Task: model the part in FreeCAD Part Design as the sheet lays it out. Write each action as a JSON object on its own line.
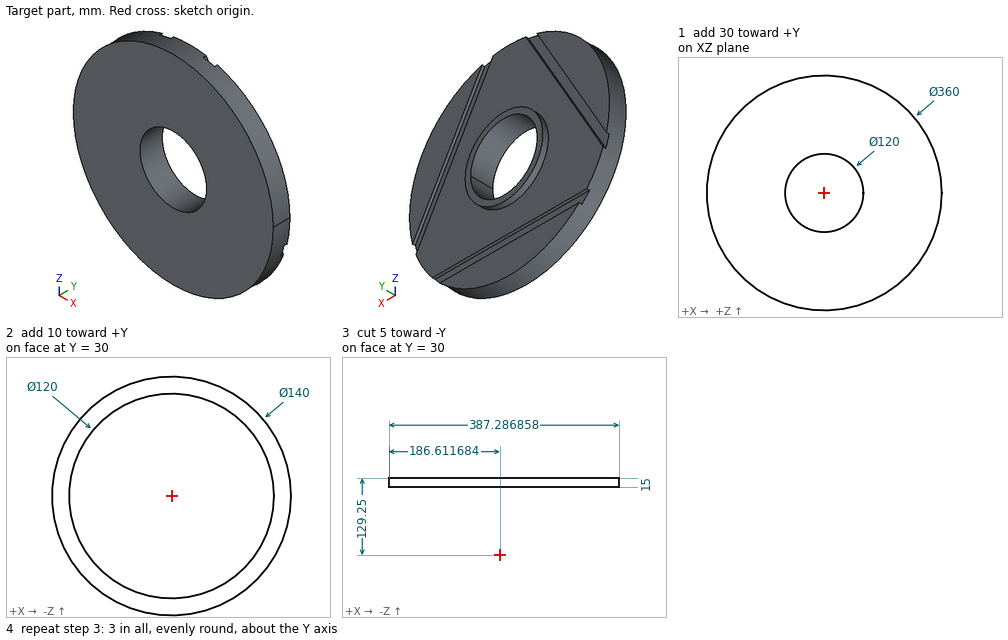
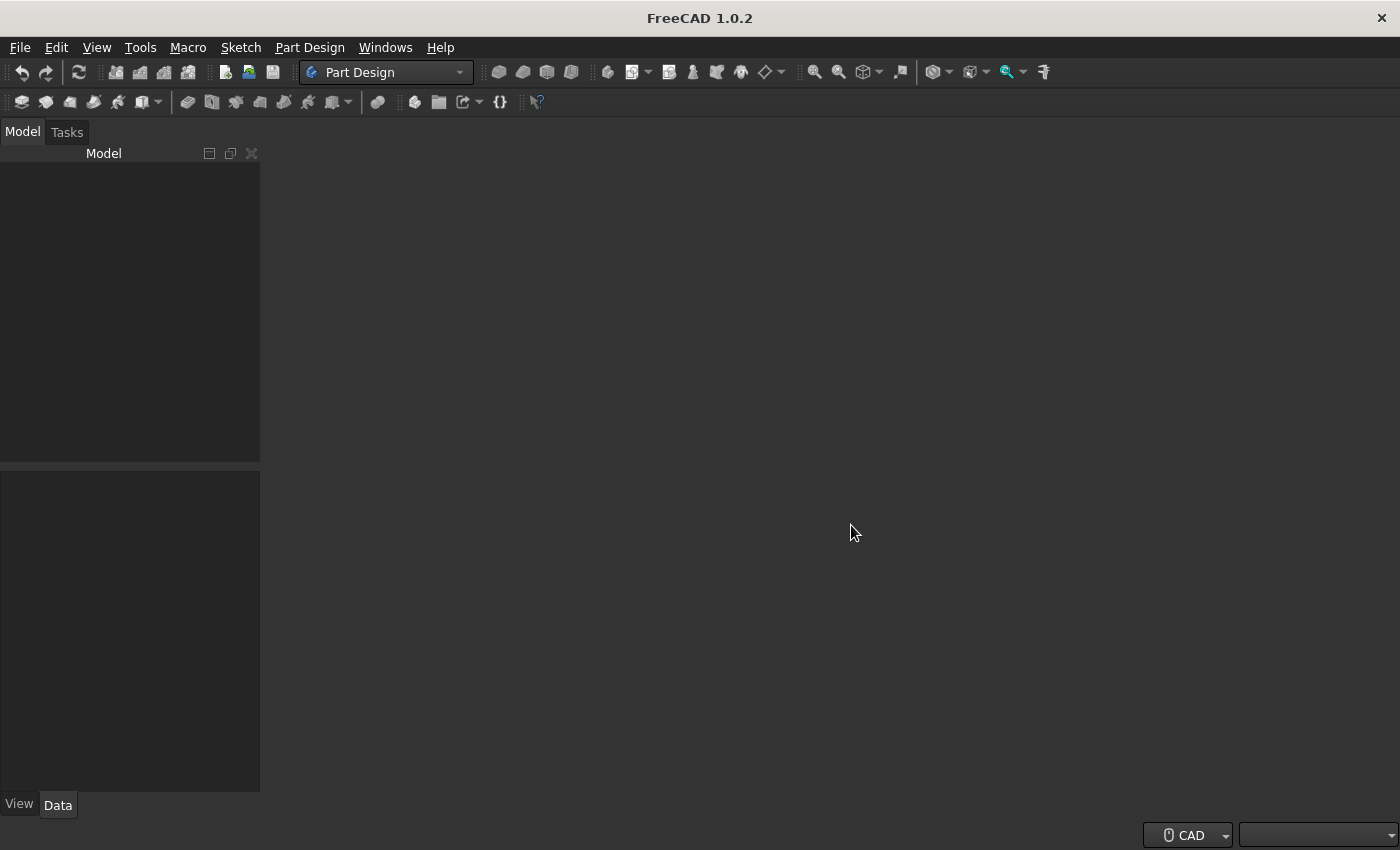
{"action": "left_click", "coordinate": [226, 72]}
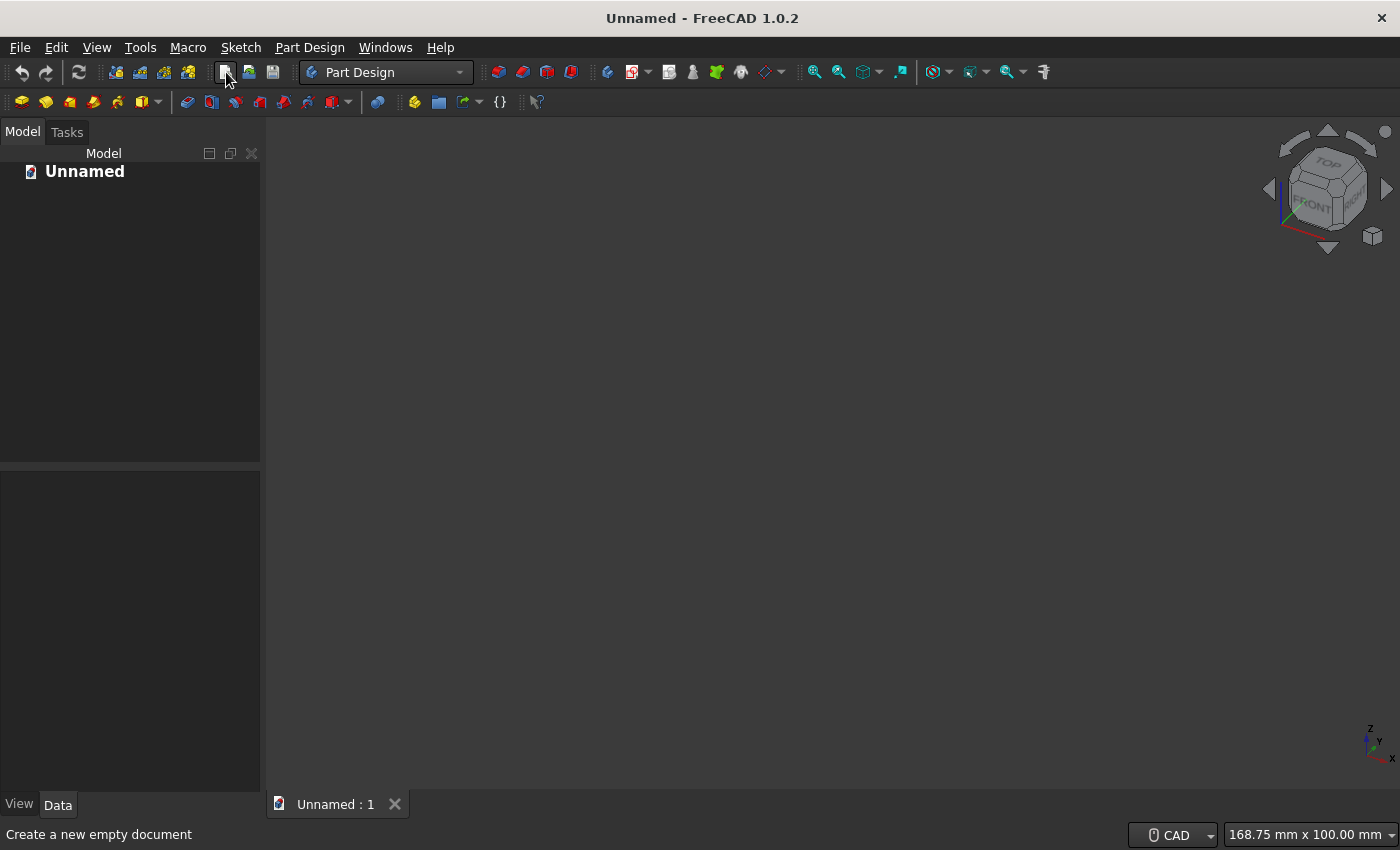
{"action": "left_click", "coordinate": [632, 72]}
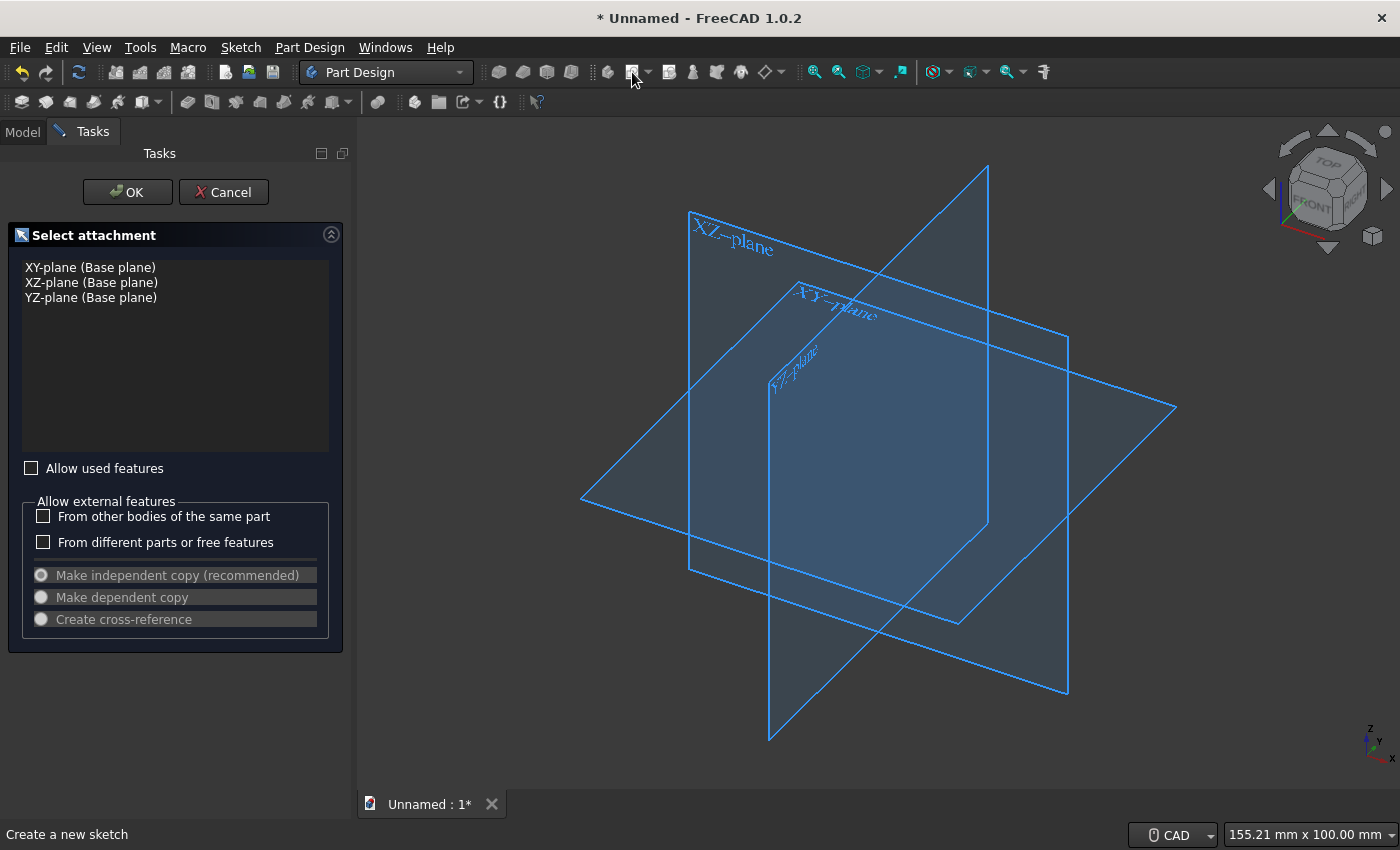
{"action": "left_click", "coordinate": [82, 282]}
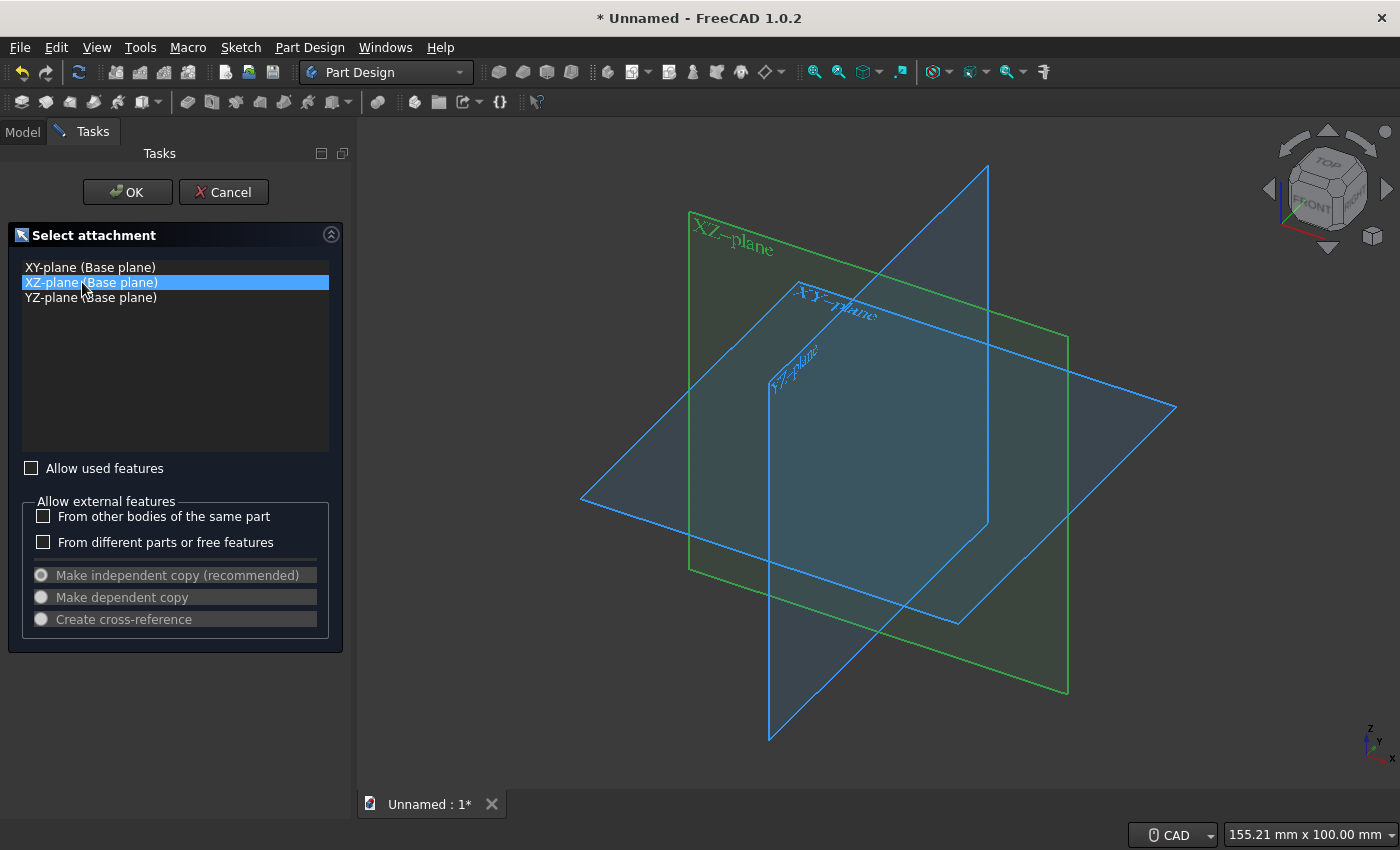
{"action": "left_click", "coordinate": [128, 192]}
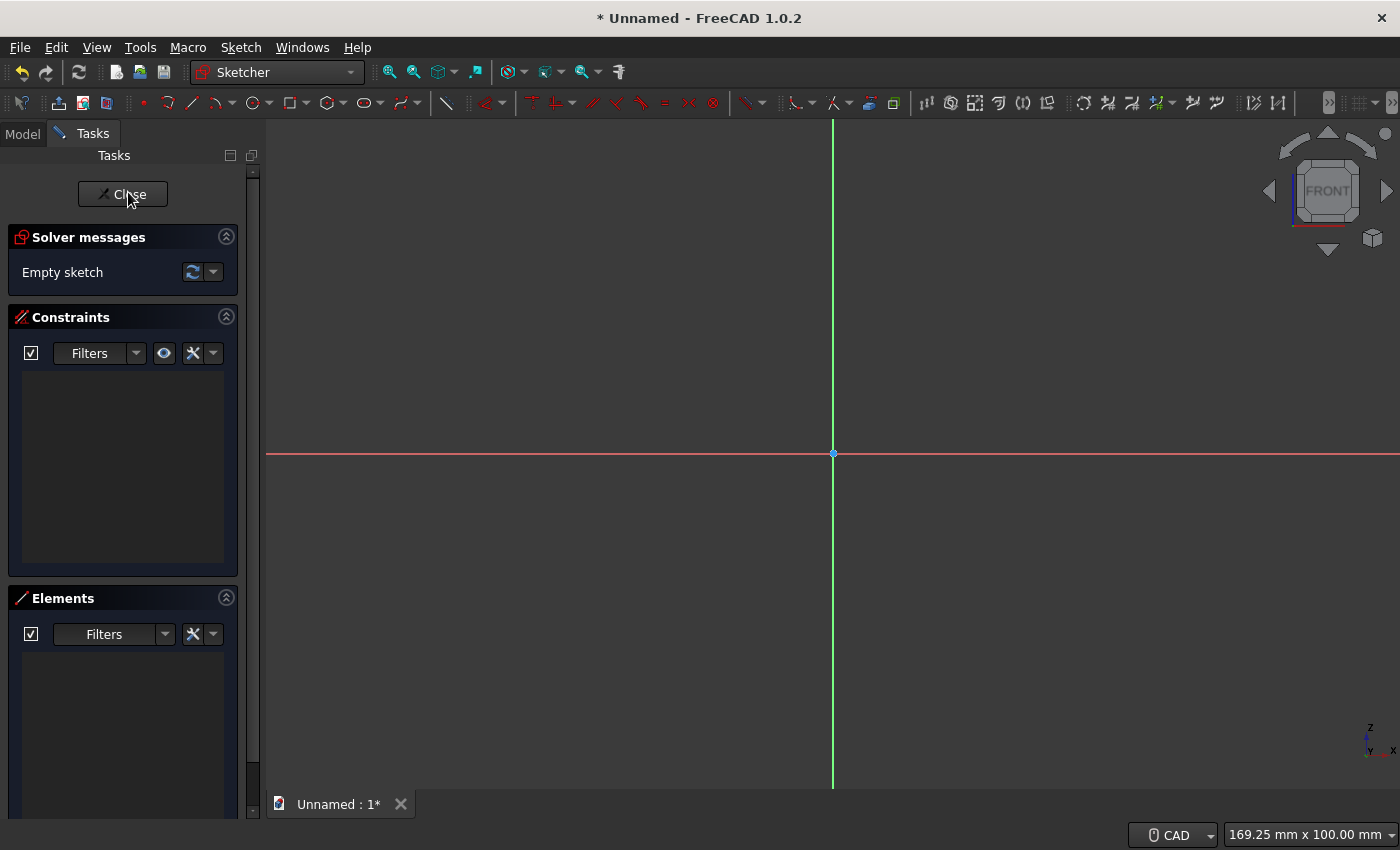
{"action": "scroll", "coordinate": [751, 454], "scroll_direction": "down", "scroll_amount": 9}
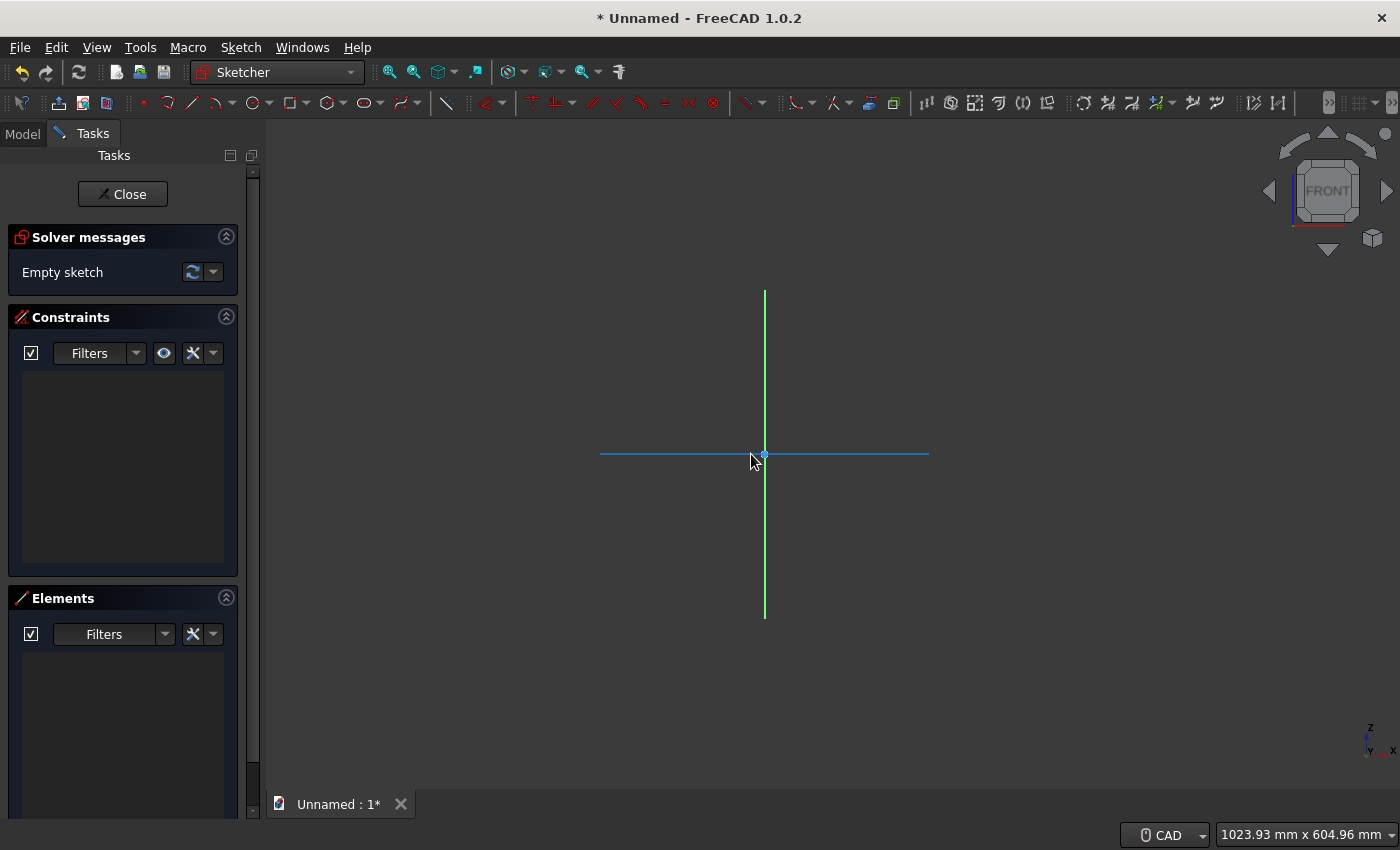
{"action": "left_click", "coordinate": [254, 104]}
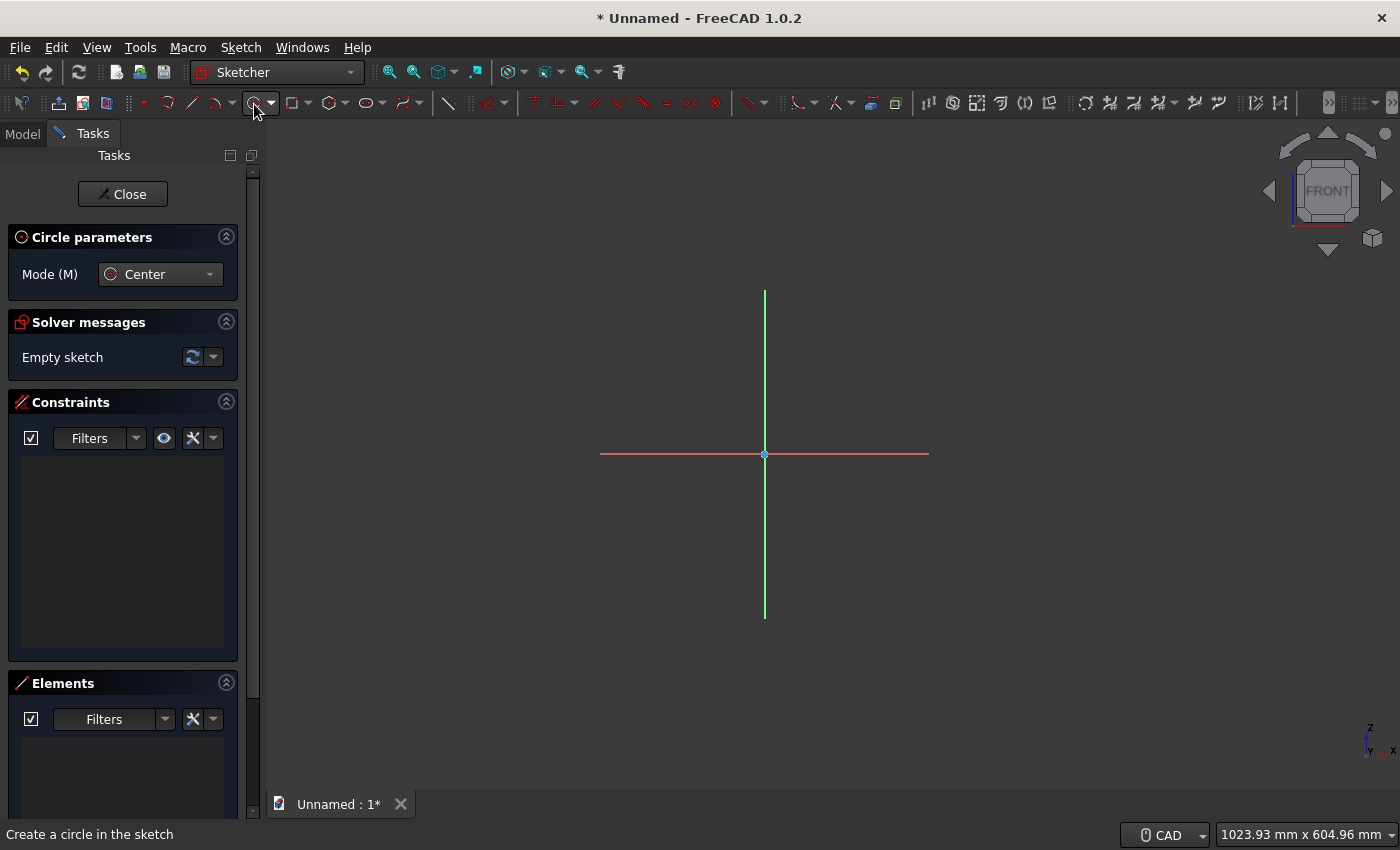
{"action": "left_click", "coordinate": [765, 454]}
{"action": "mouse_move", "coordinate": [906, 313]}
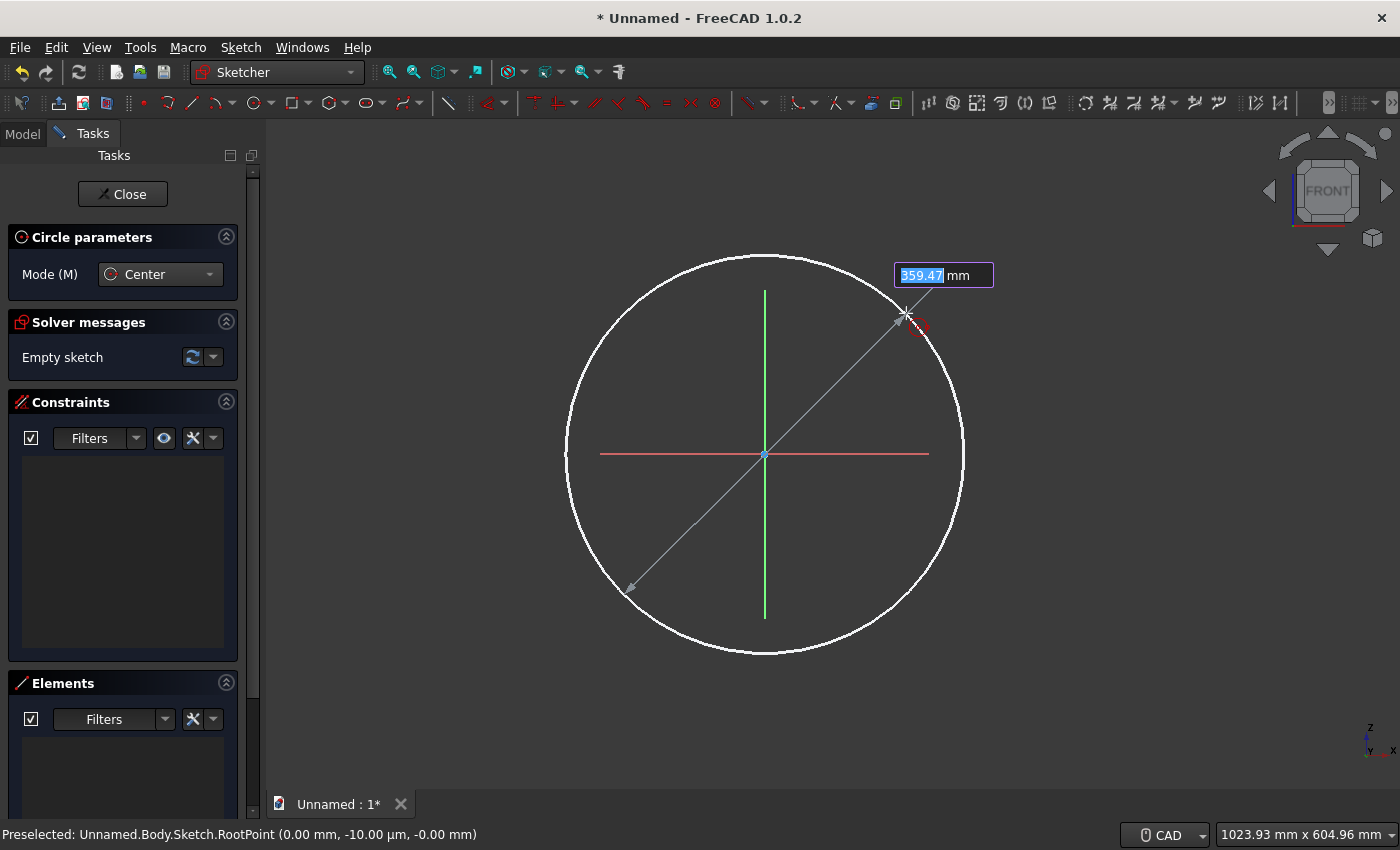
{"action": "type", "text": "360"}
{"action": "key", "text": "Return"}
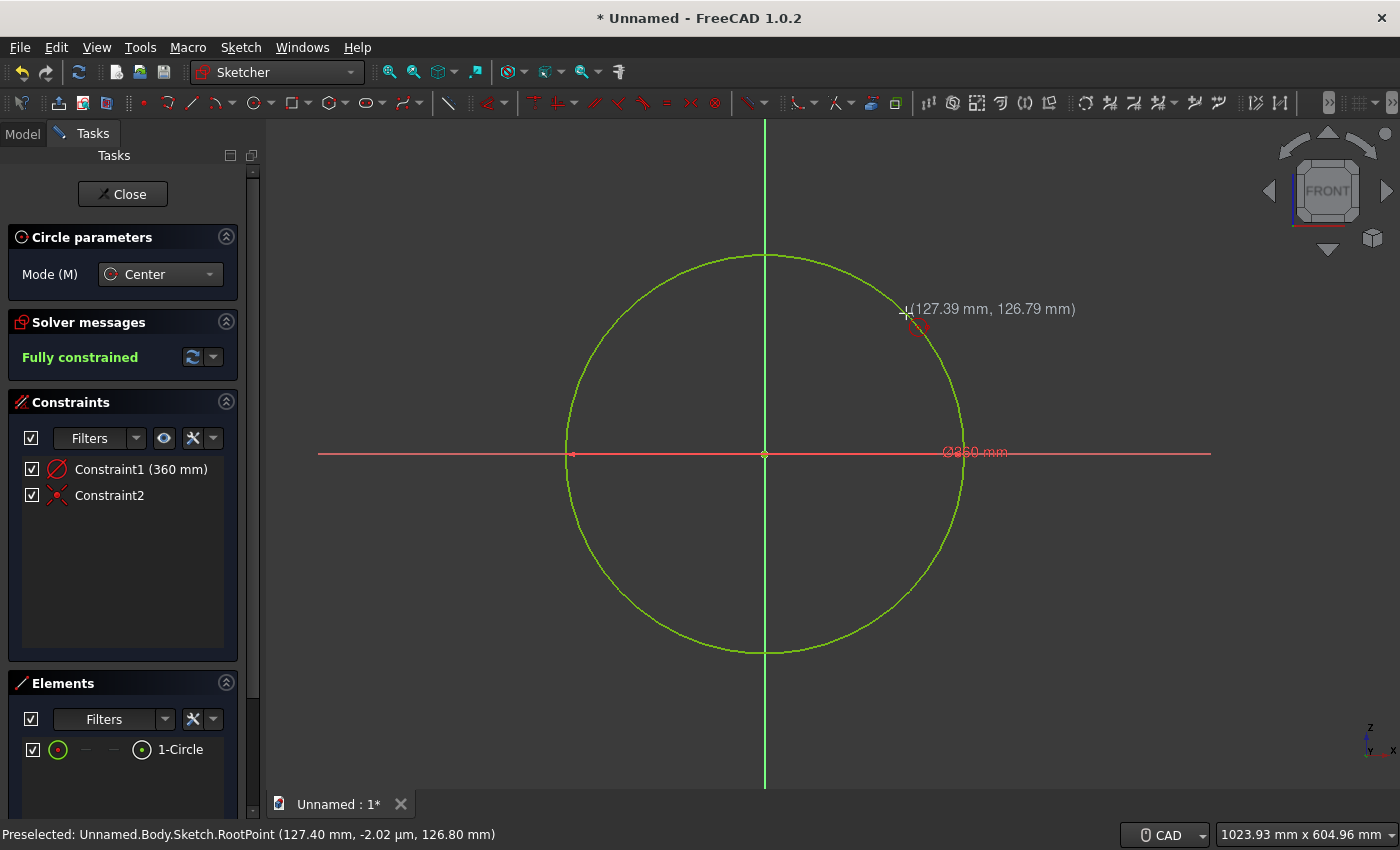
{"action": "left_click", "coordinate": [765, 454]}
{"action": "mouse_move", "coordinate": [812, 407]}